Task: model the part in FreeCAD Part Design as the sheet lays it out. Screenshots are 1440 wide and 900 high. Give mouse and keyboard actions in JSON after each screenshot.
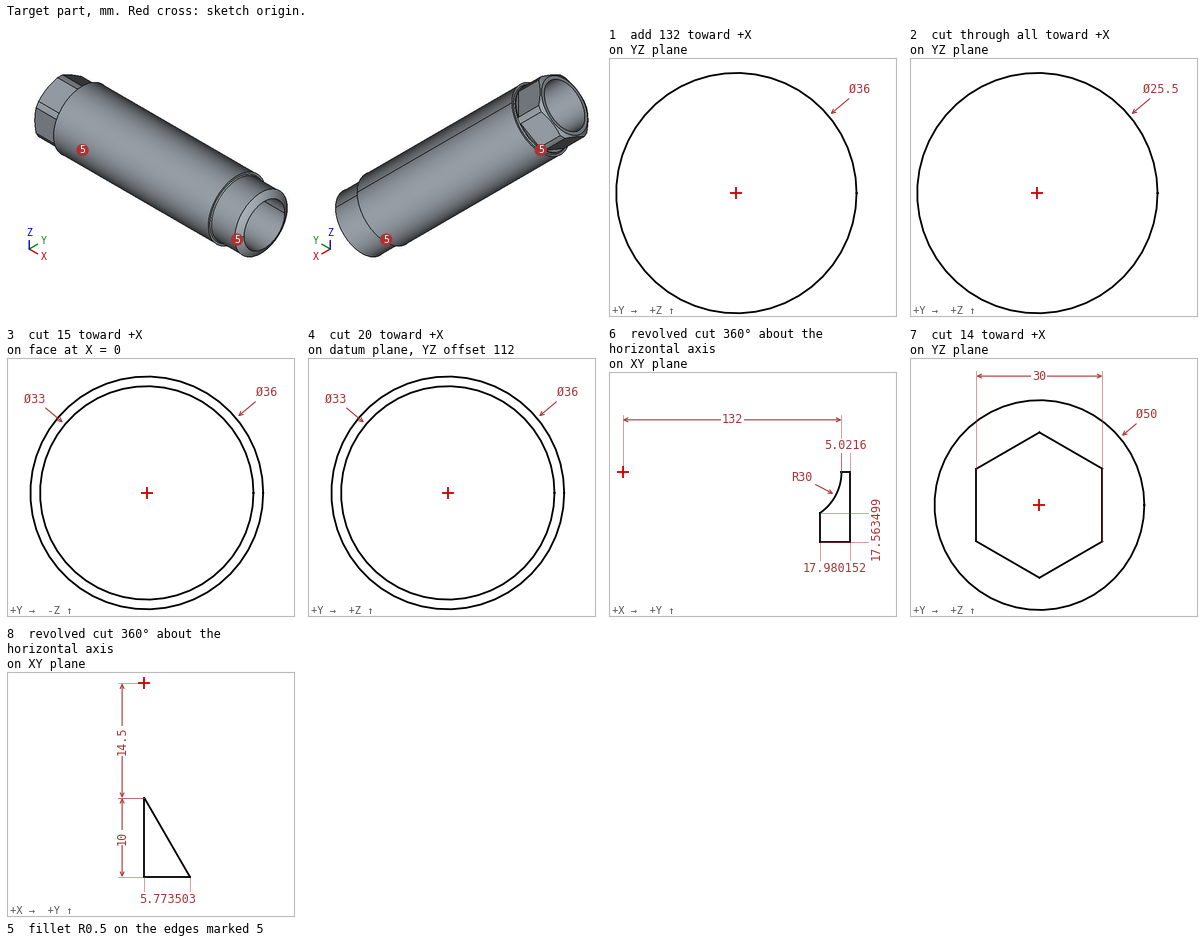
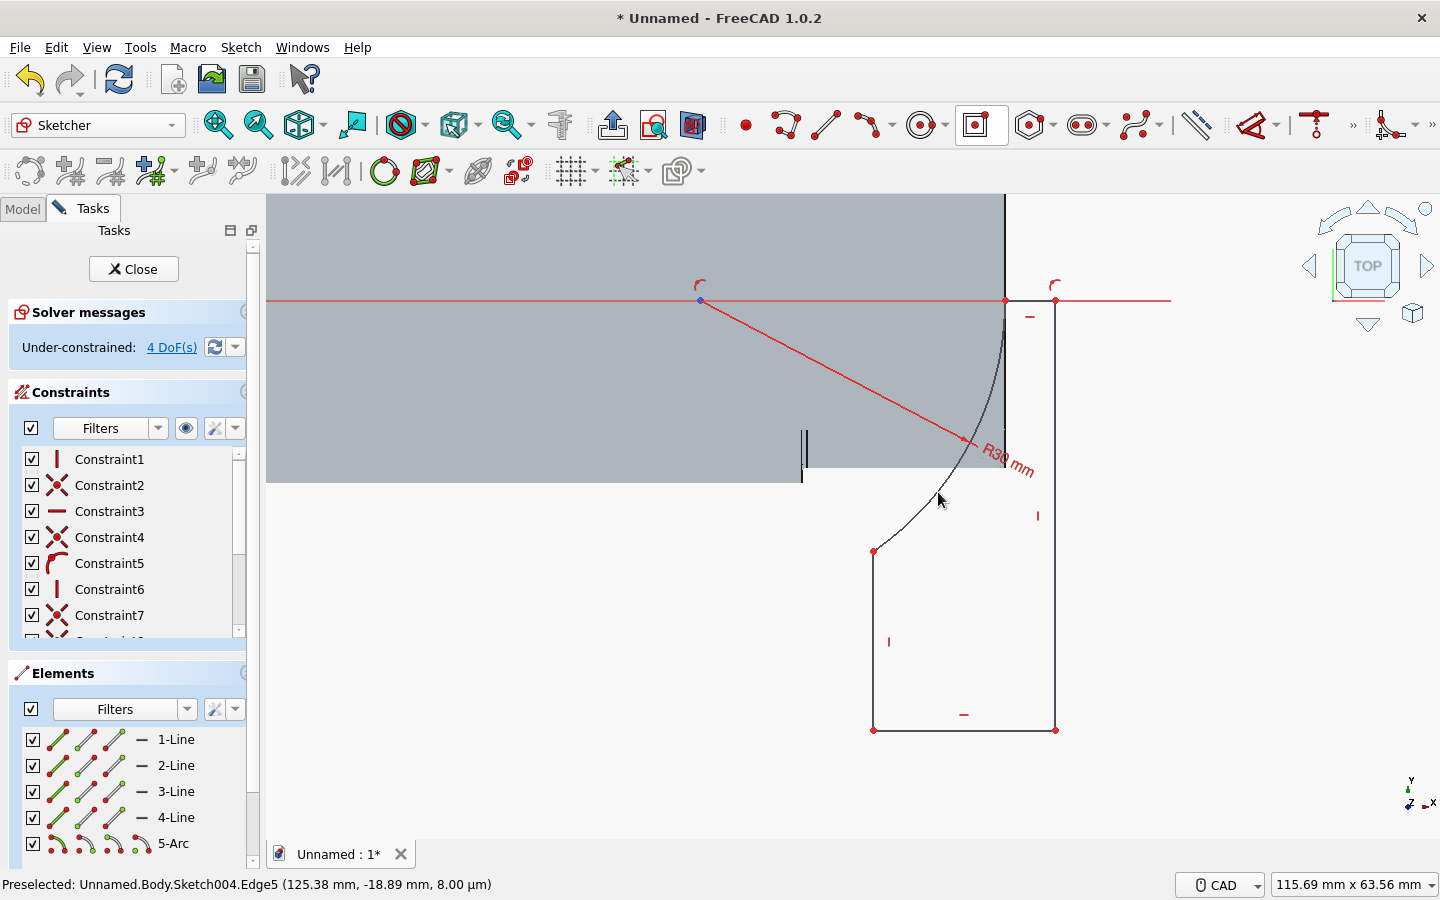
{"action": "left_click", "coordinate": [1005, 301]}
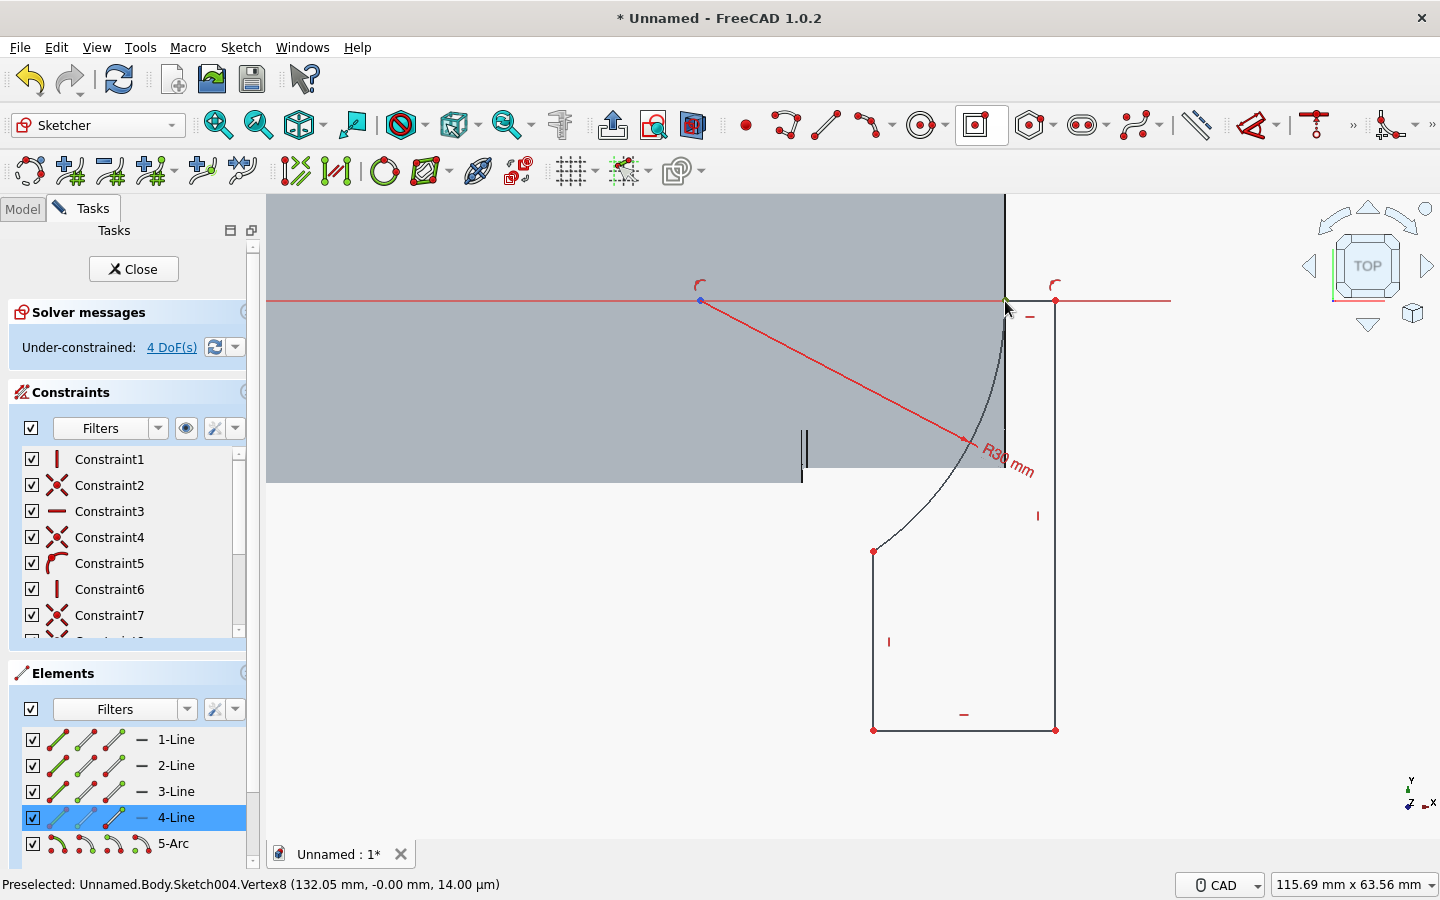
{"action": "left_click", "coordinate": [1278, 126]}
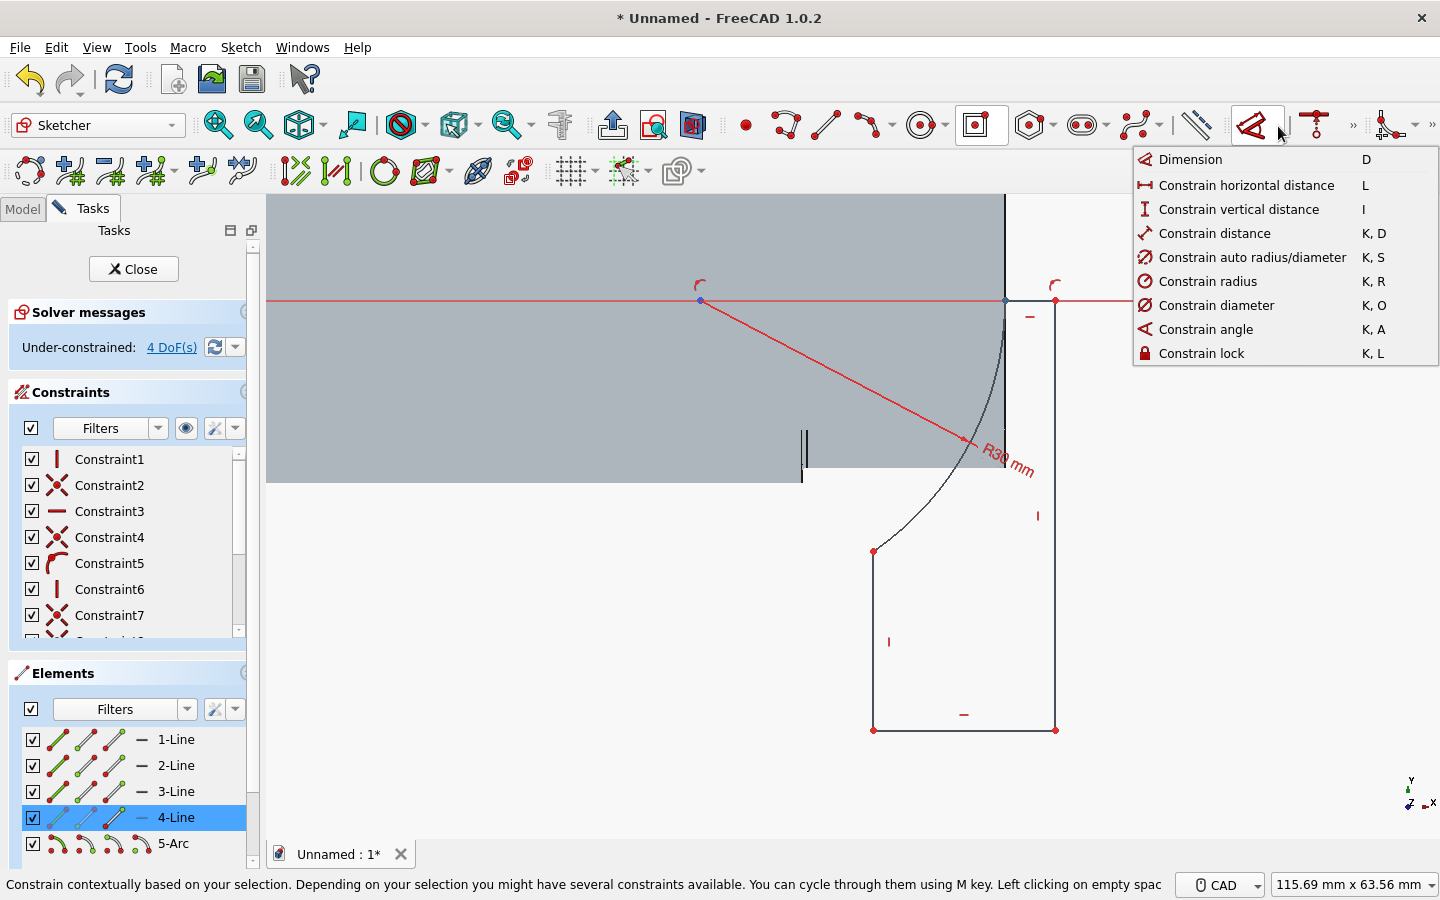
{"action": "left_click", "coordinate": [1286, 185]}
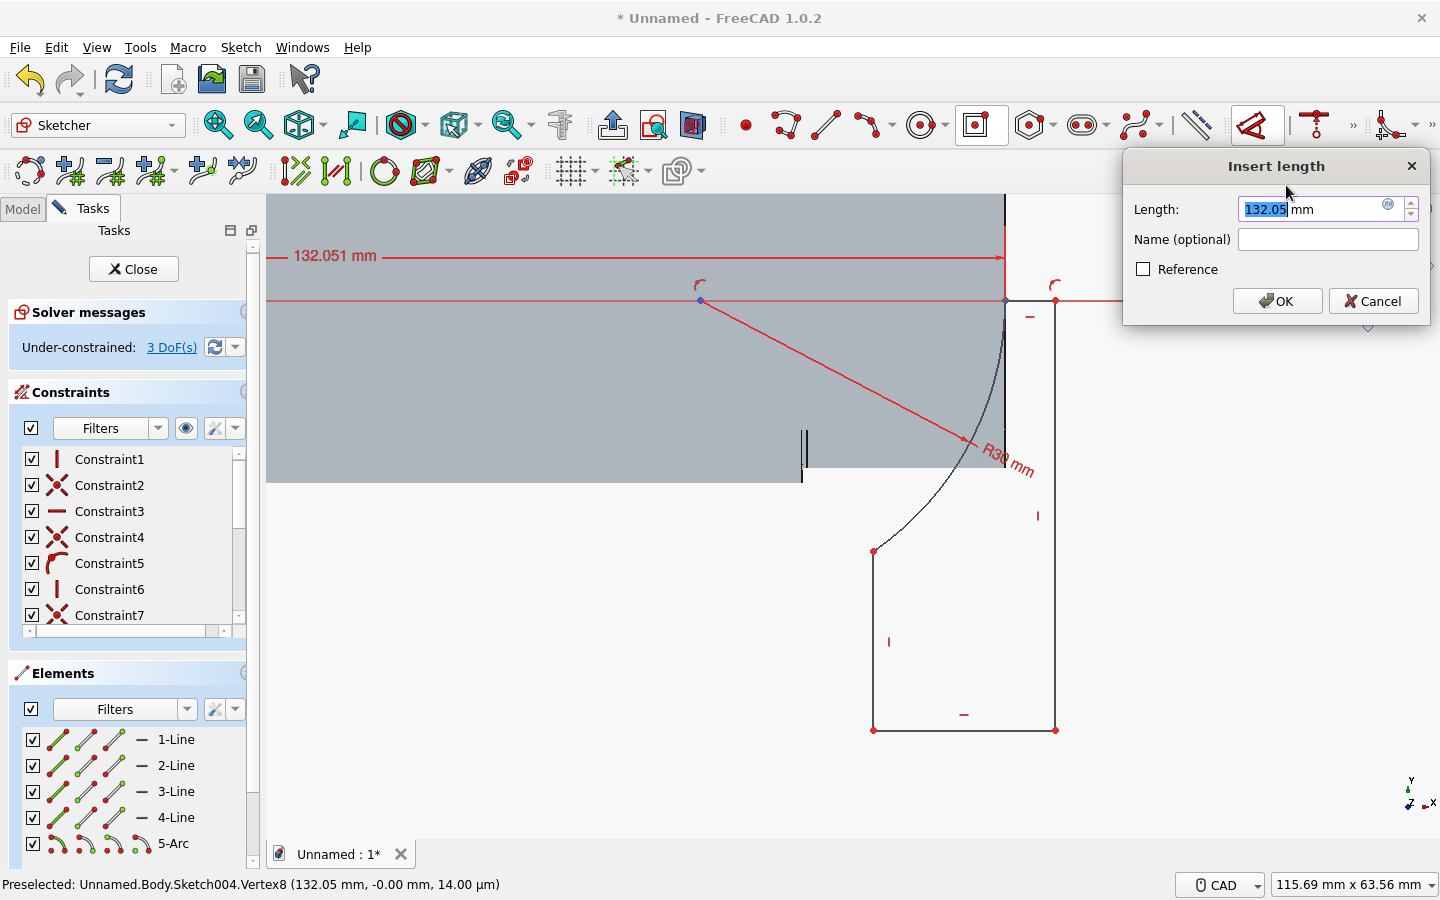
{"action": "type", "text": "132"}
{"action": "key", "text": "Return"}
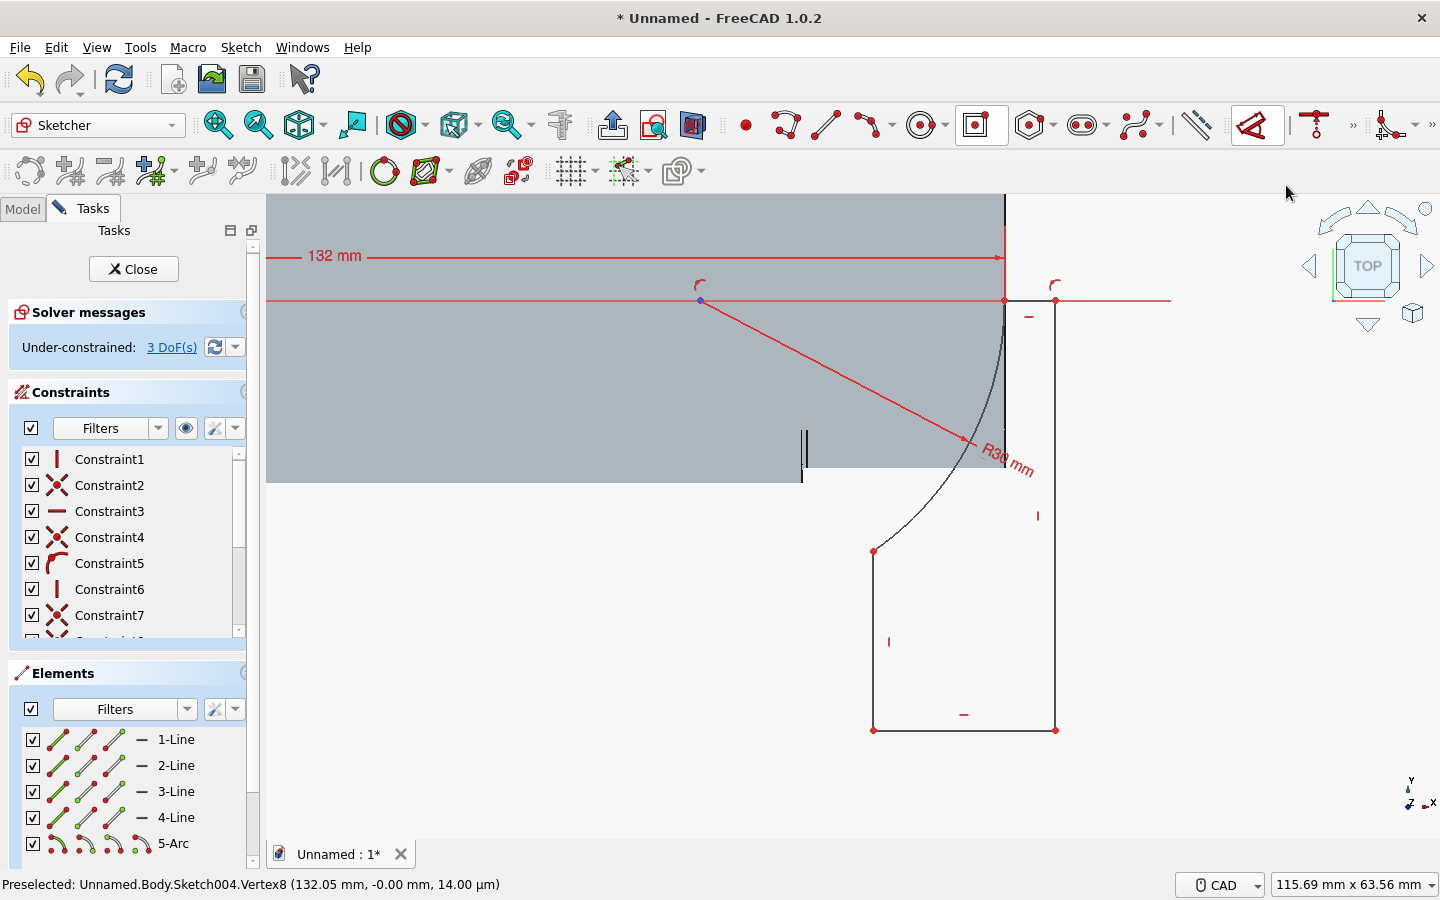
{"action": "left_click", "coordinate": [1040, 301]}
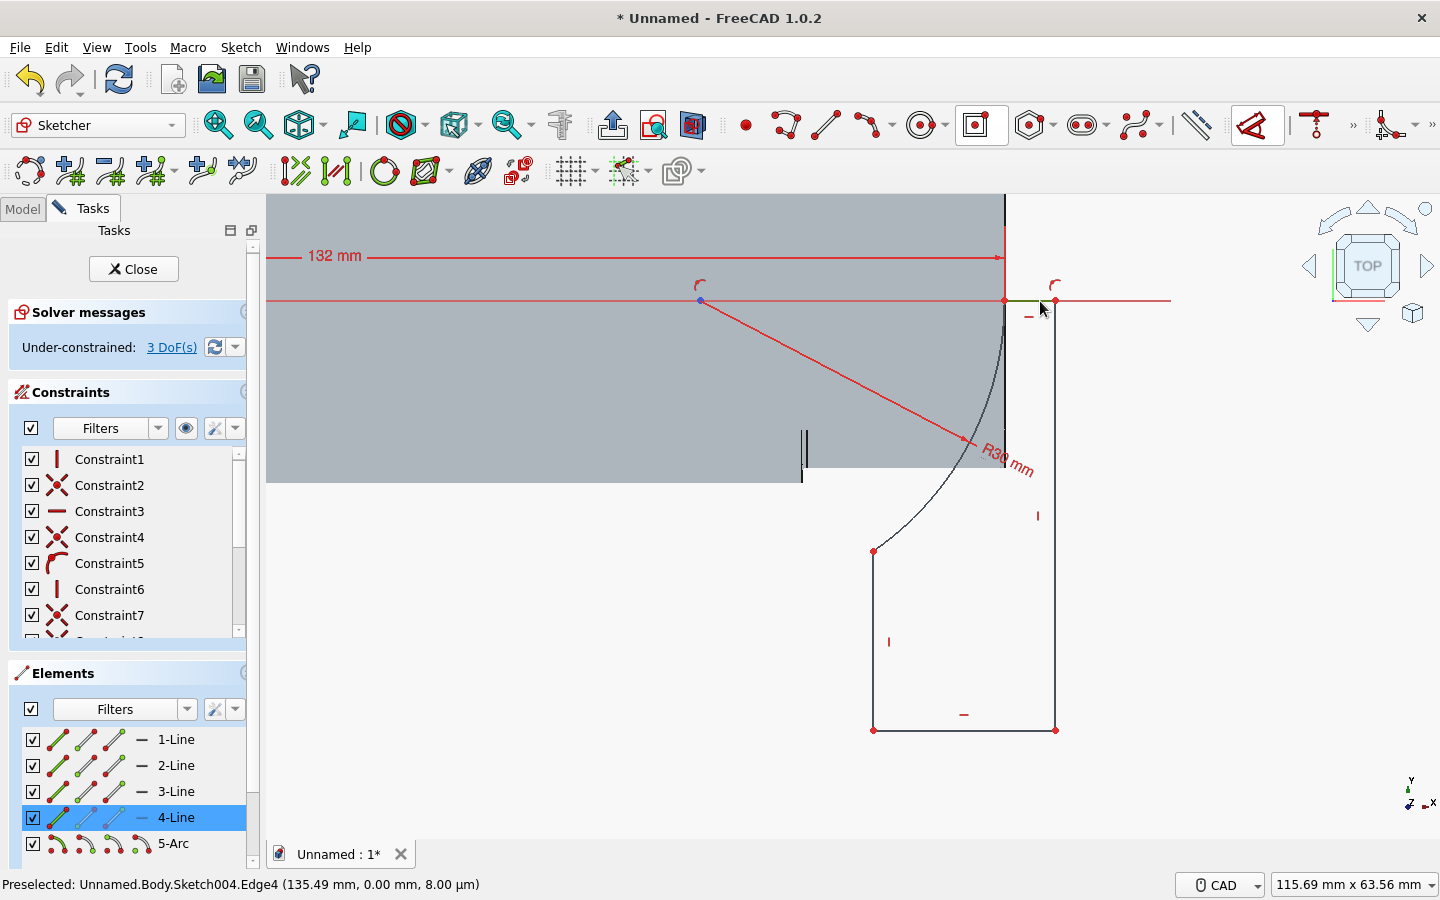
{"action": "left_click", "coordinate": [1278, 126]}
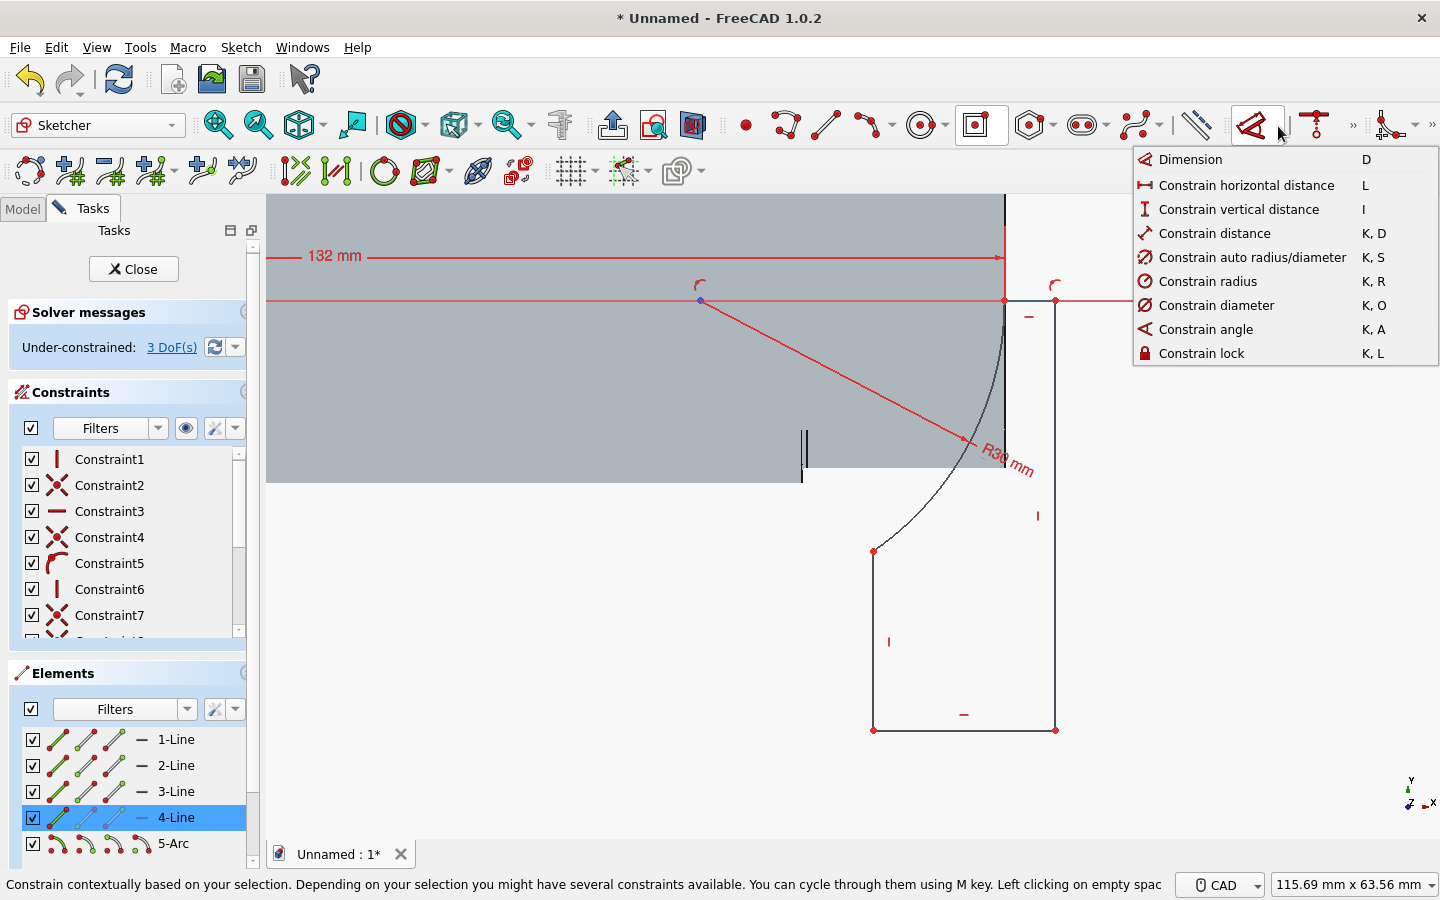
{"action": "left_click", "coordinate": [1286, 185]}